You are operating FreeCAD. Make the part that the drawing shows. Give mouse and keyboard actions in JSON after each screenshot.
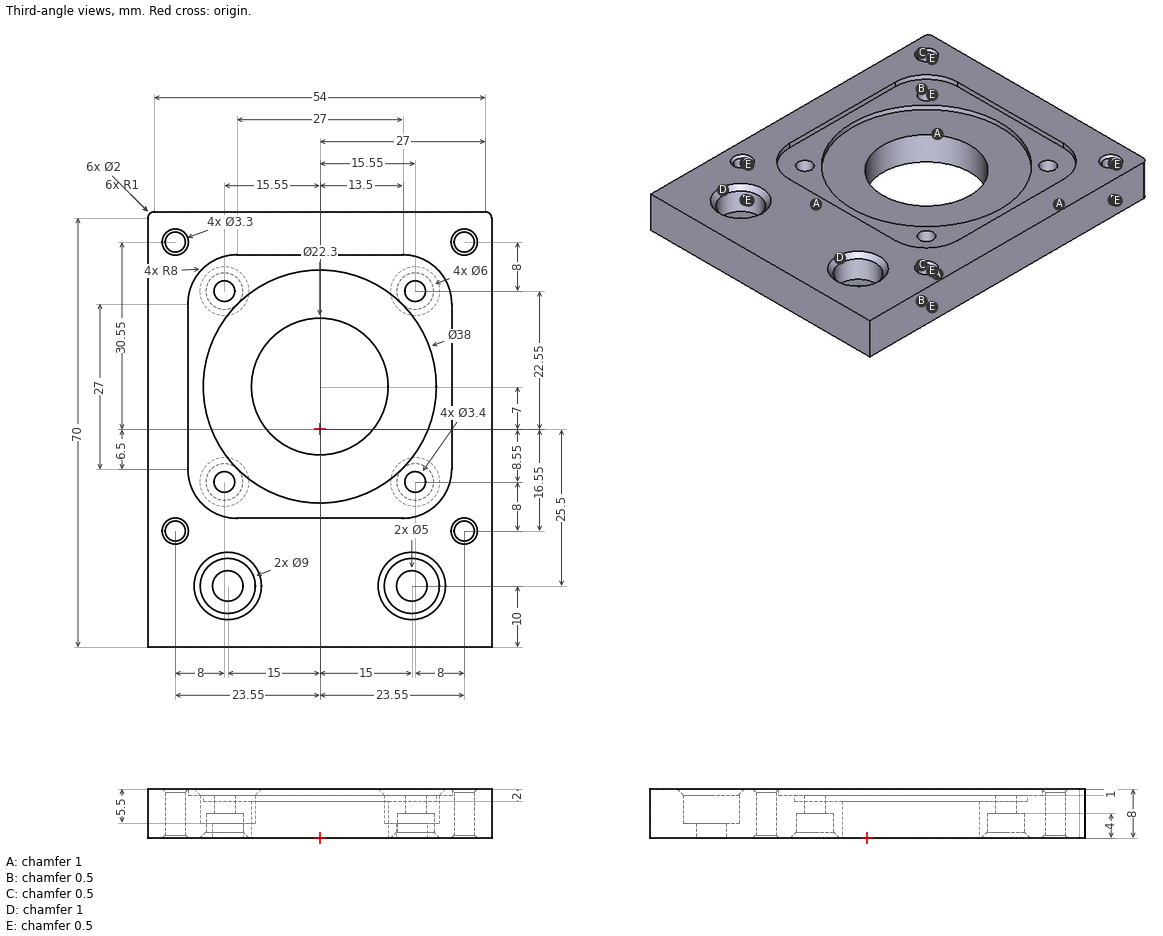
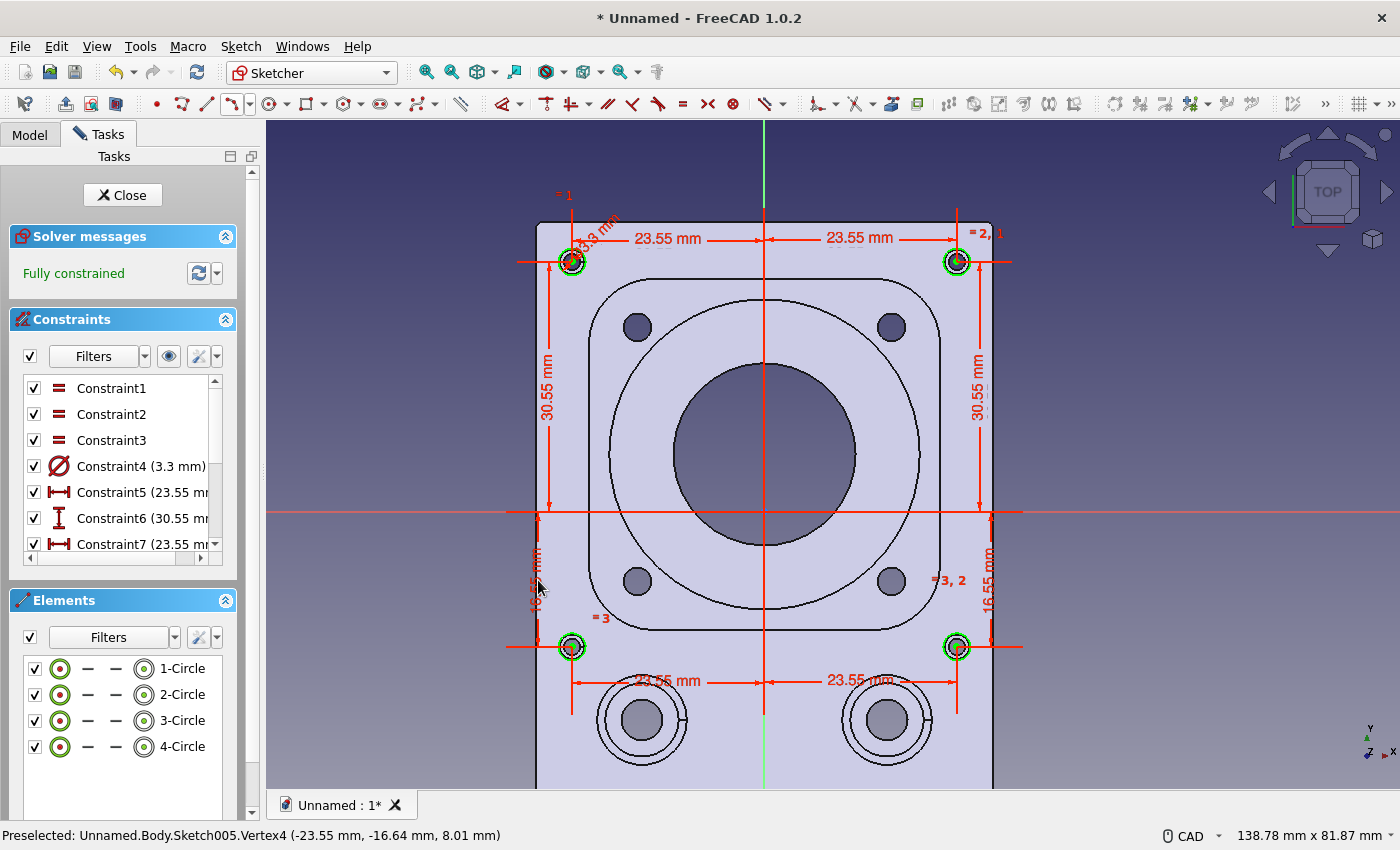
{"action": "left_click", "coordinate": [123, 195]}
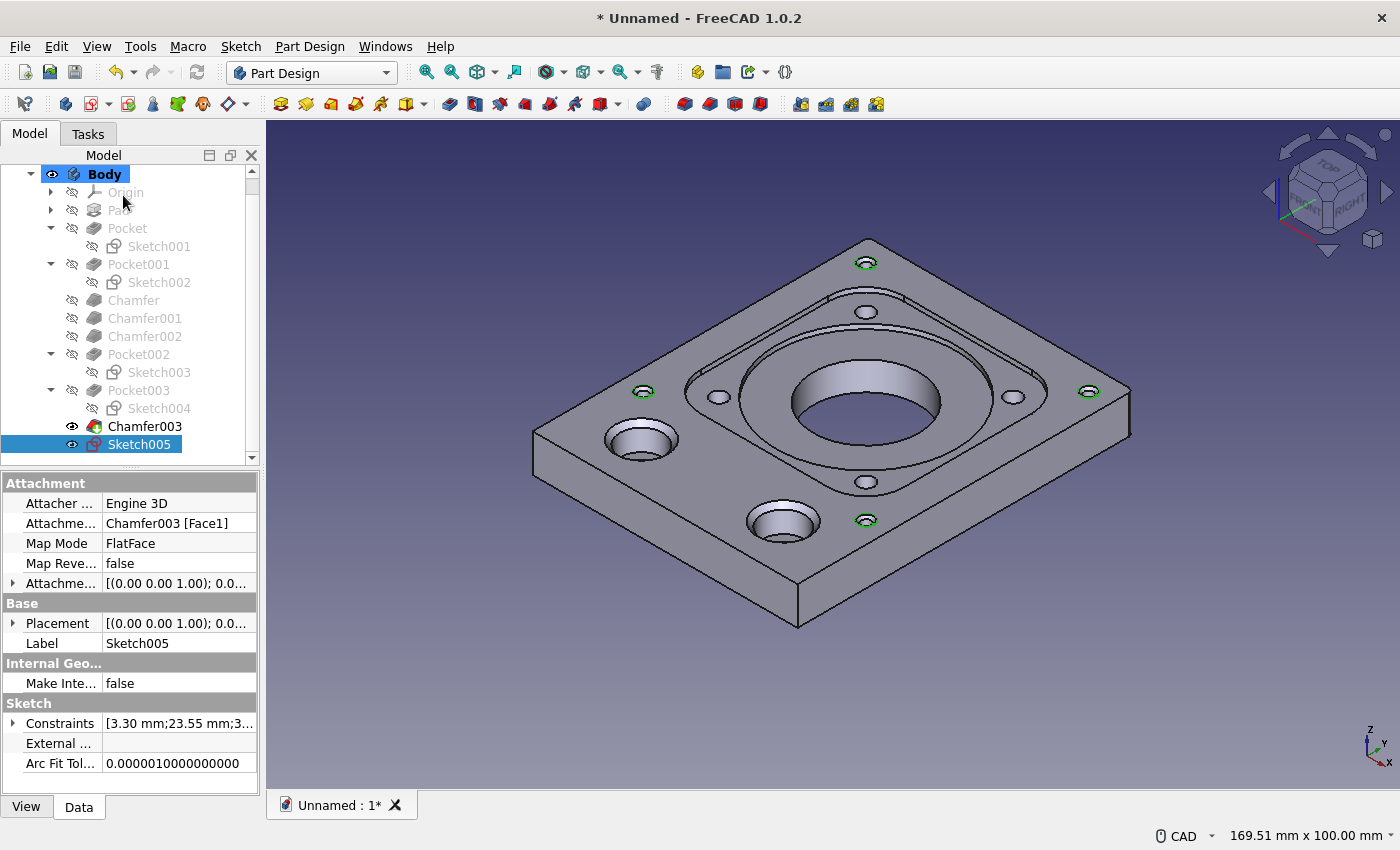
{"action": "left_click", "coordinate": [450, 104]}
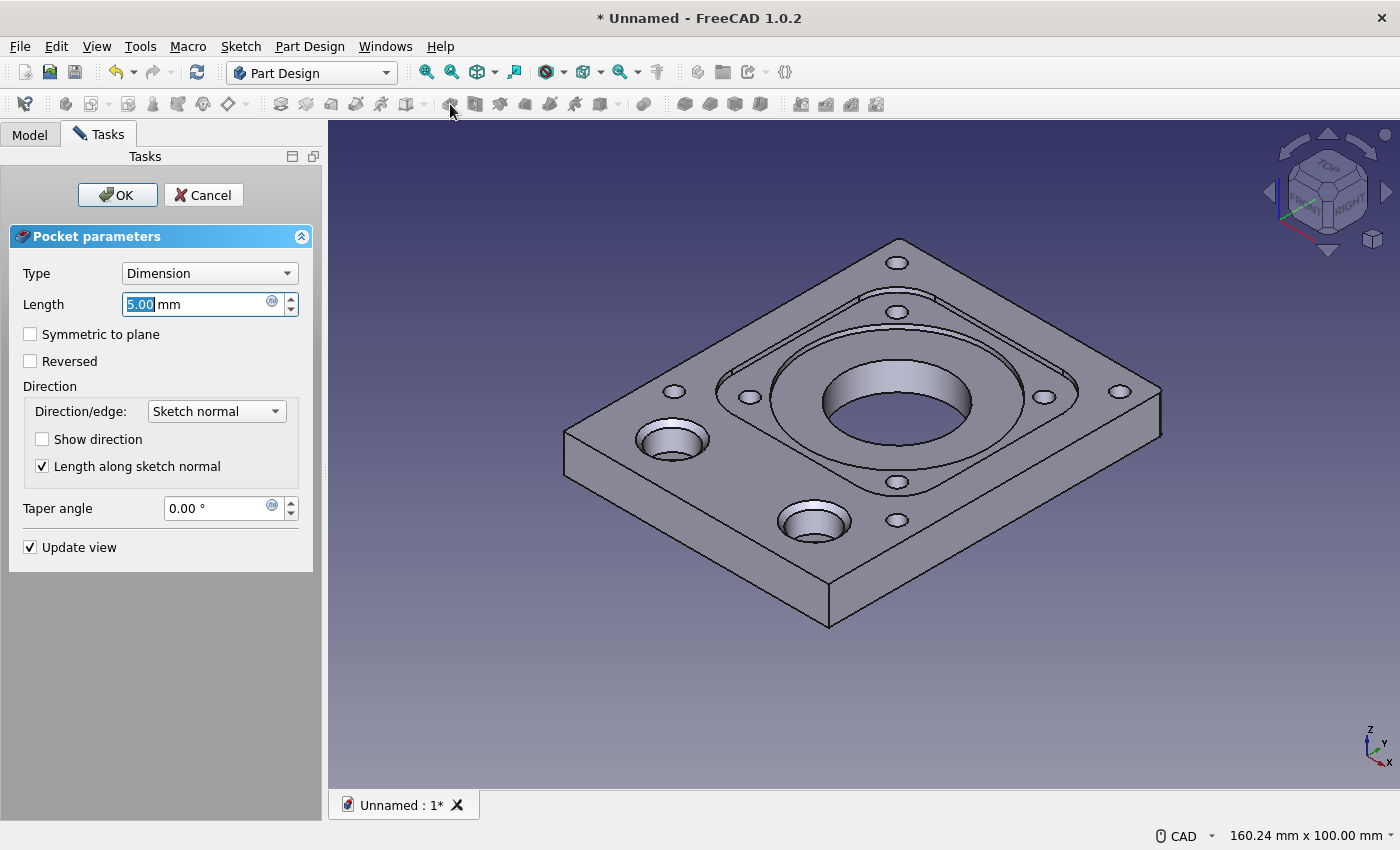
{"action": "left_click", "coordinate": [210, 274]}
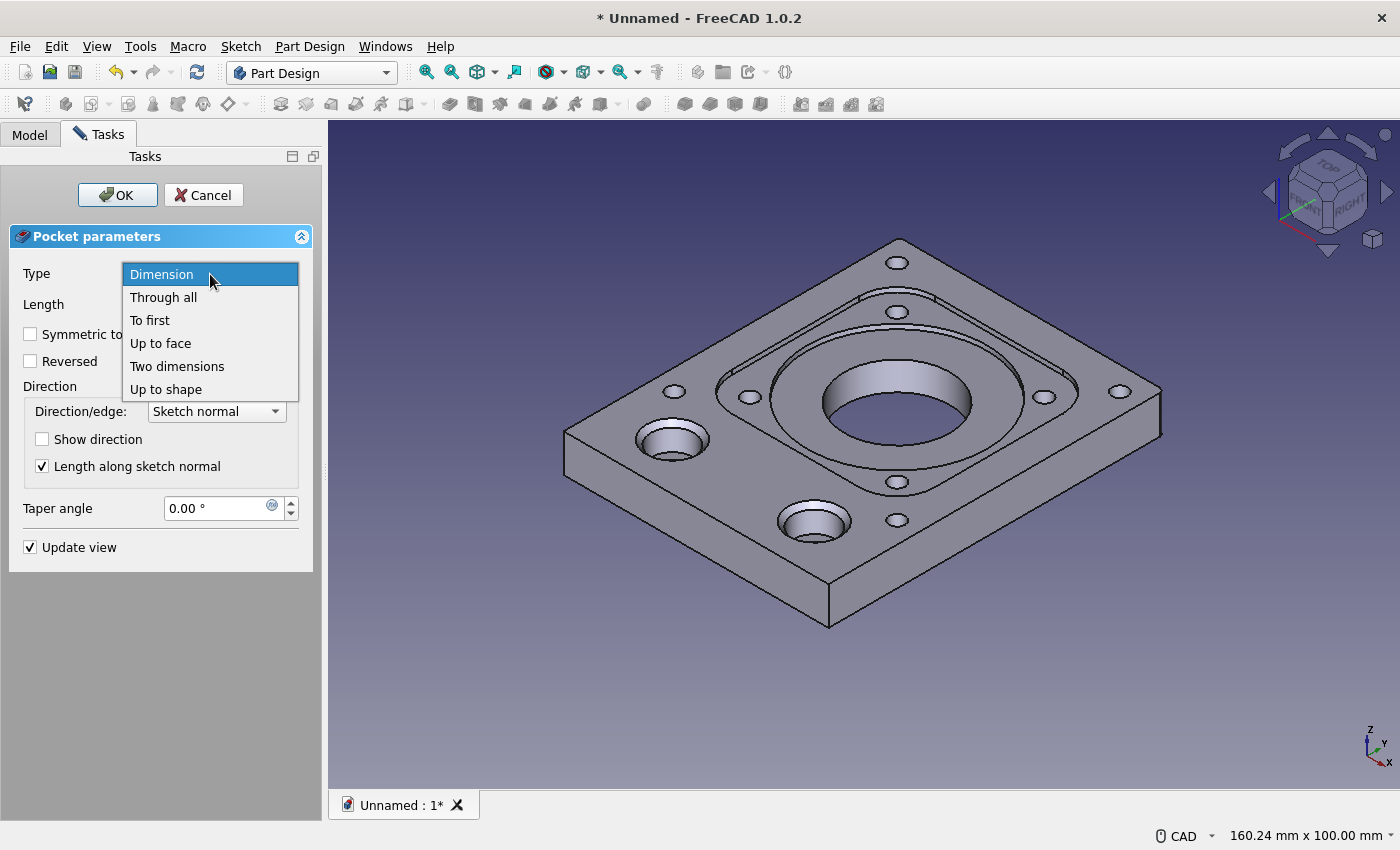
{"action": "left_click", "coordinate": [208, 298]}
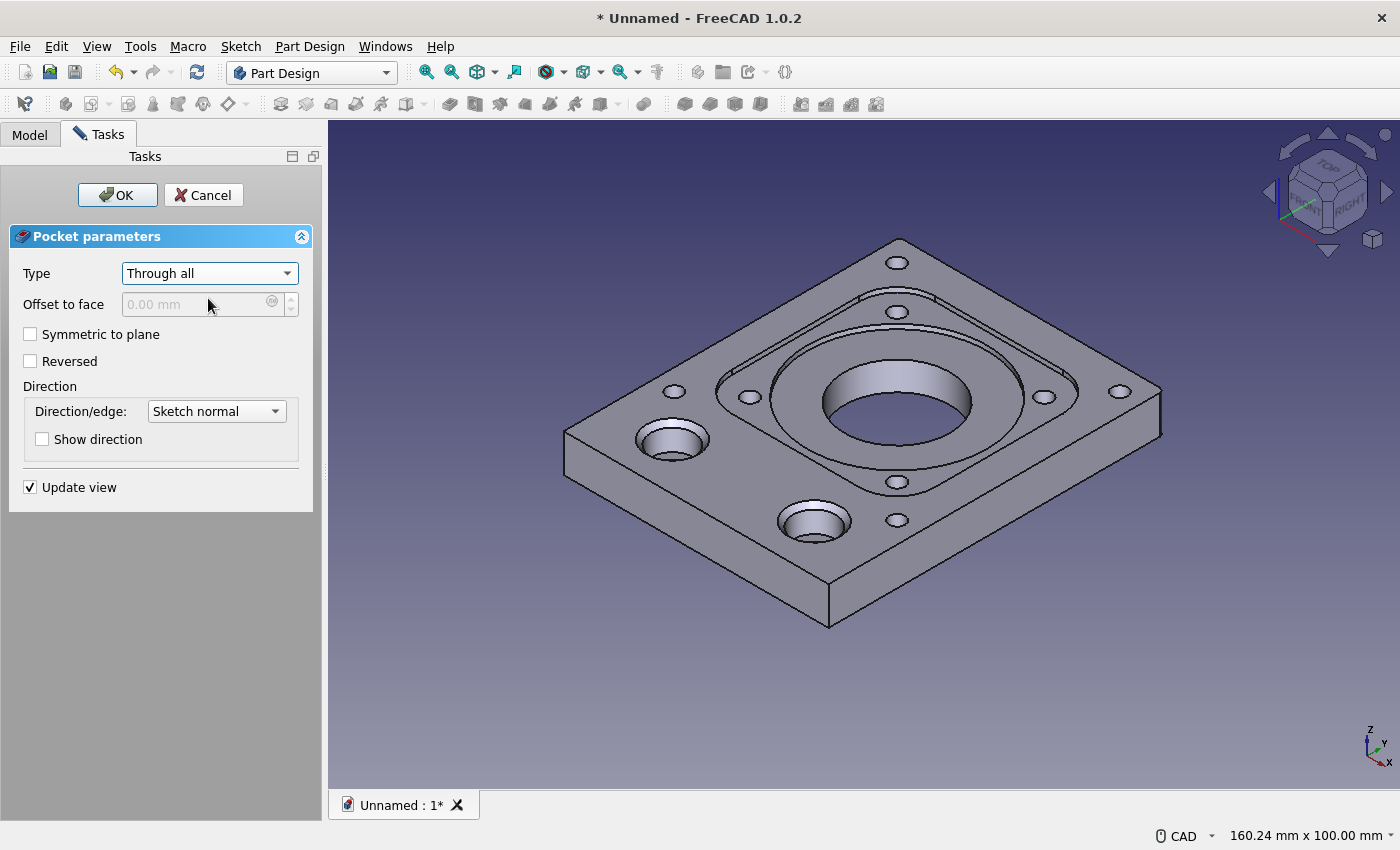
{"action": "left_click", "coordinate": [118, 195]}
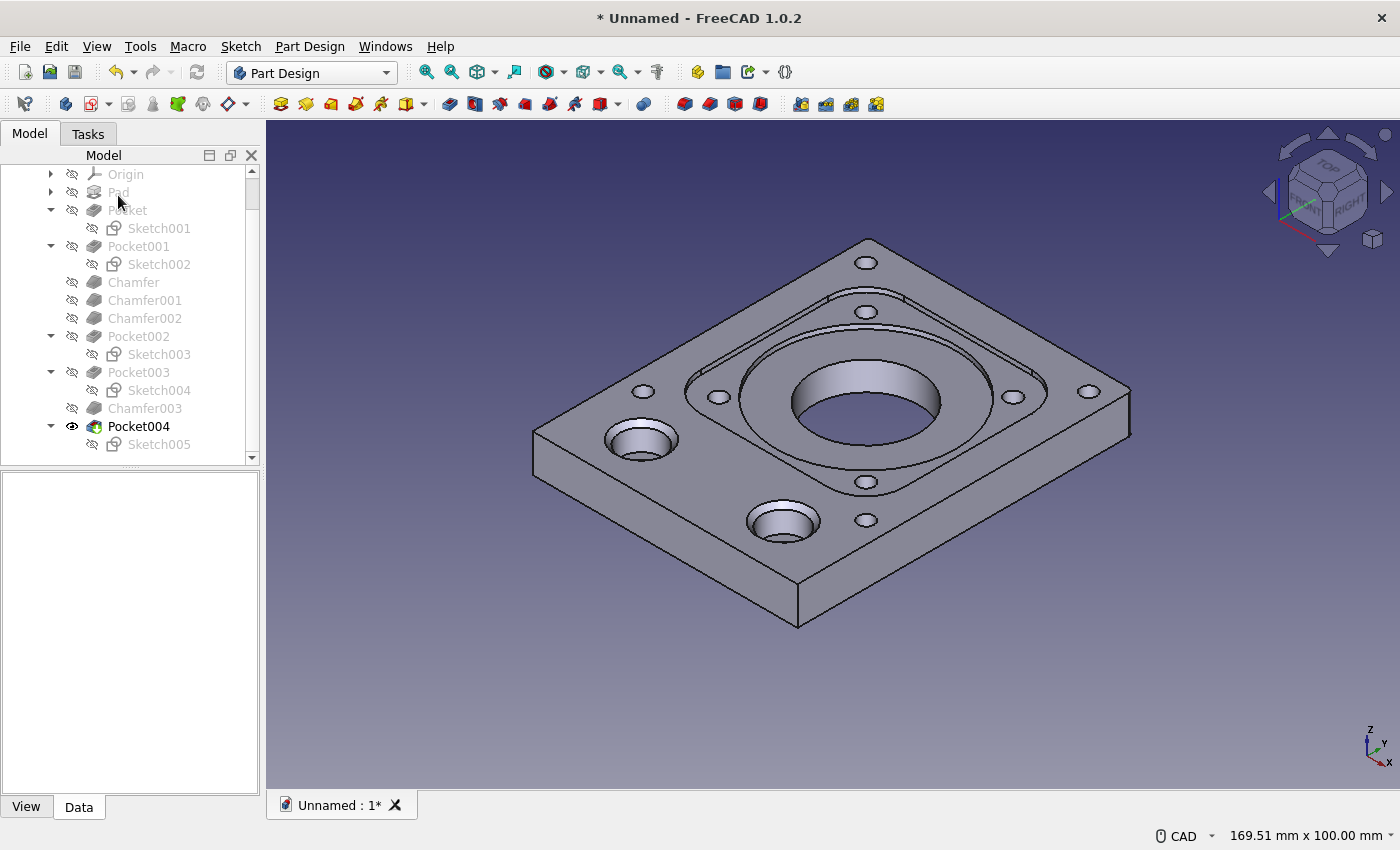
{"action": "left_click", "coordinate": [635, 386]}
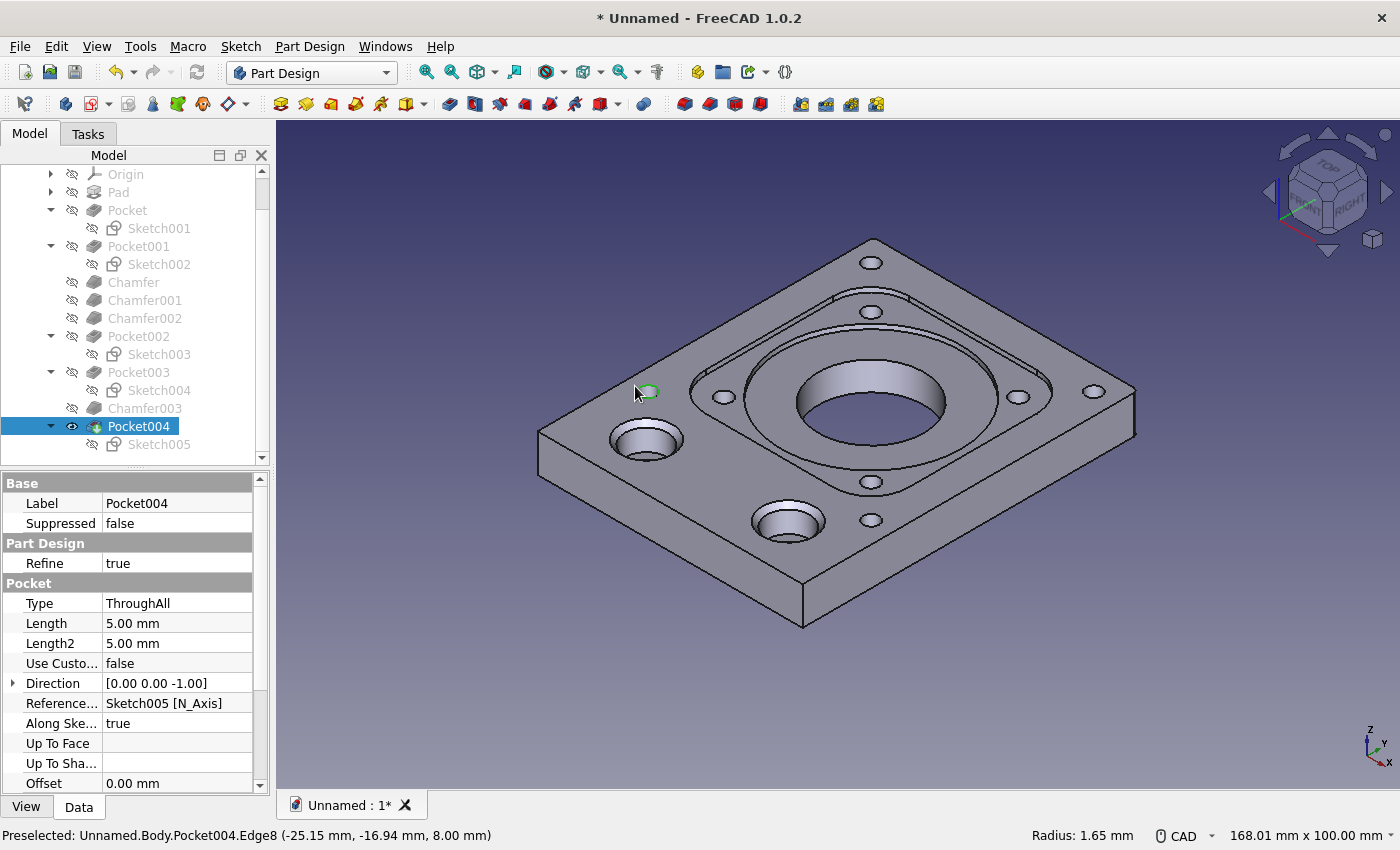
{"action": "left_click", "coordinate": [863, 515], "text": "ctrl"}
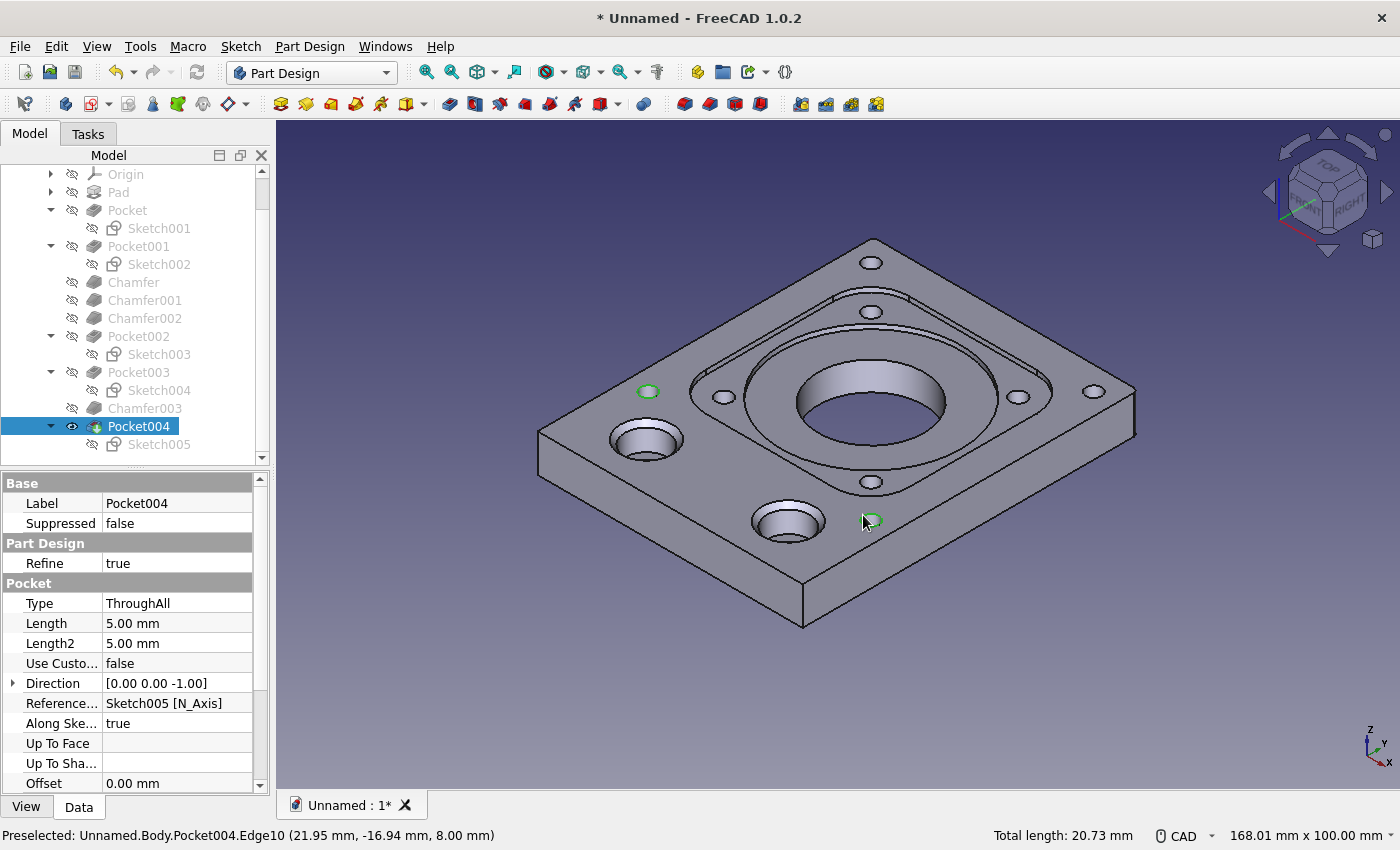
{"action": "left_click", "coordinate": [1086, 386], "text": "ctrl"}